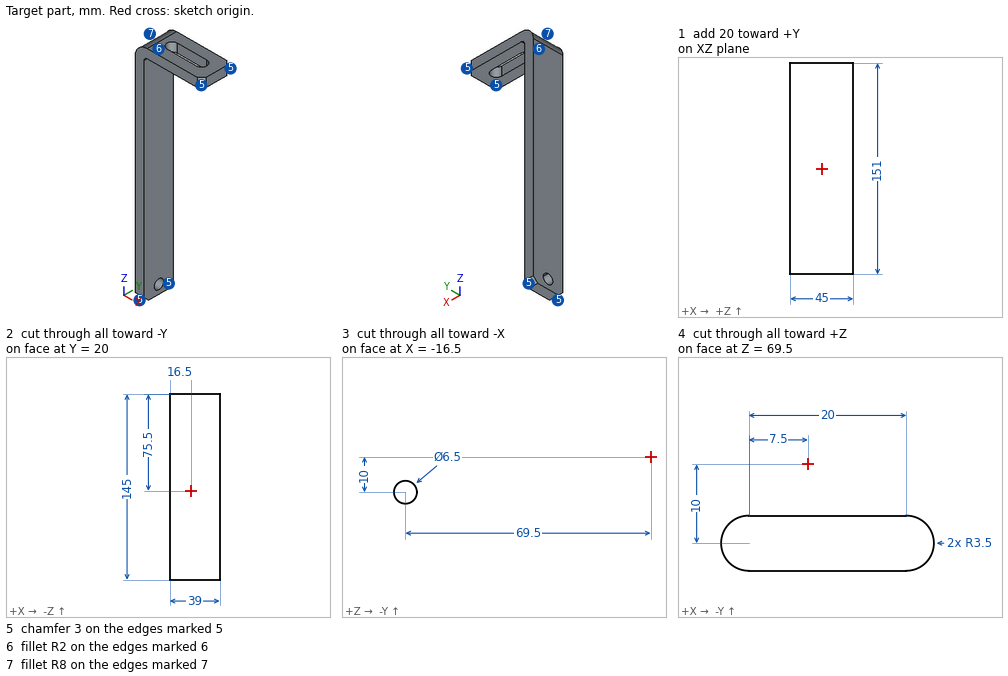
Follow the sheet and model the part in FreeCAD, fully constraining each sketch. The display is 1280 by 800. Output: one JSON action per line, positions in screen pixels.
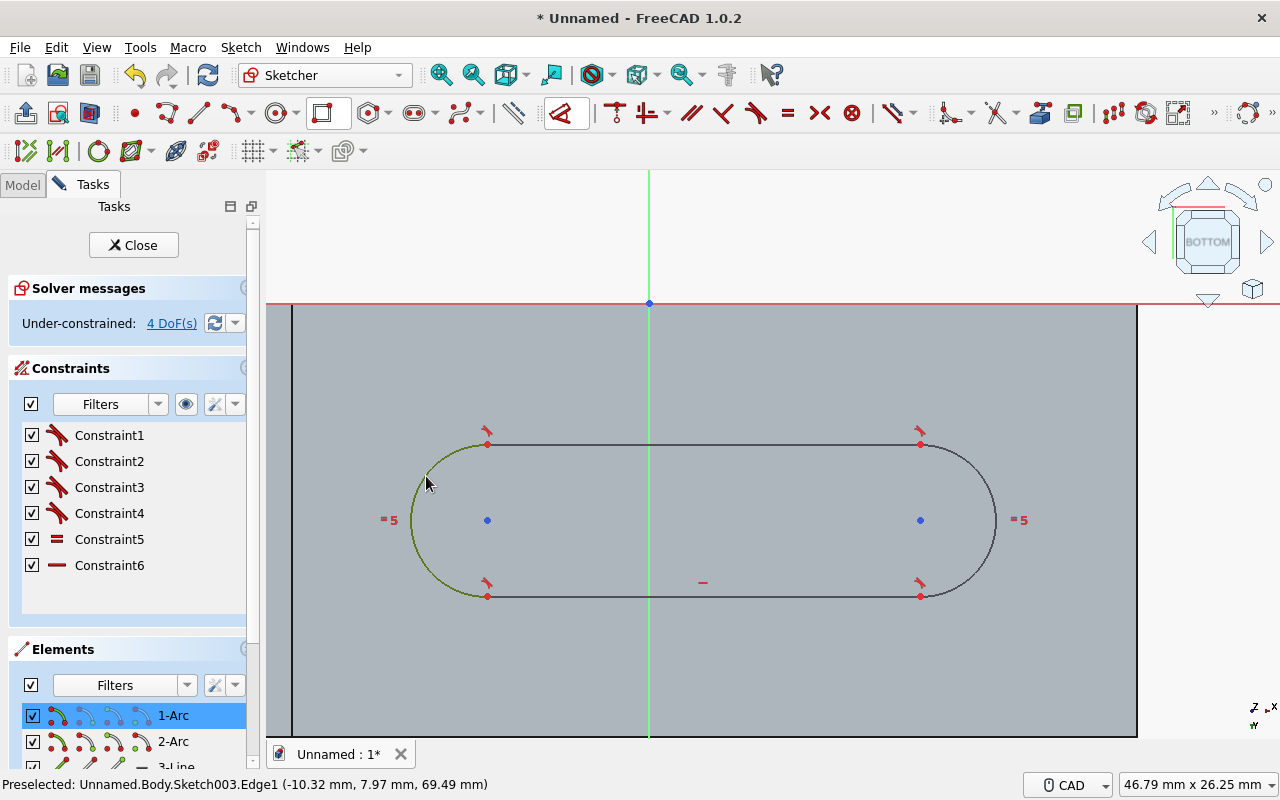
{"action": "key", "text": "k r"}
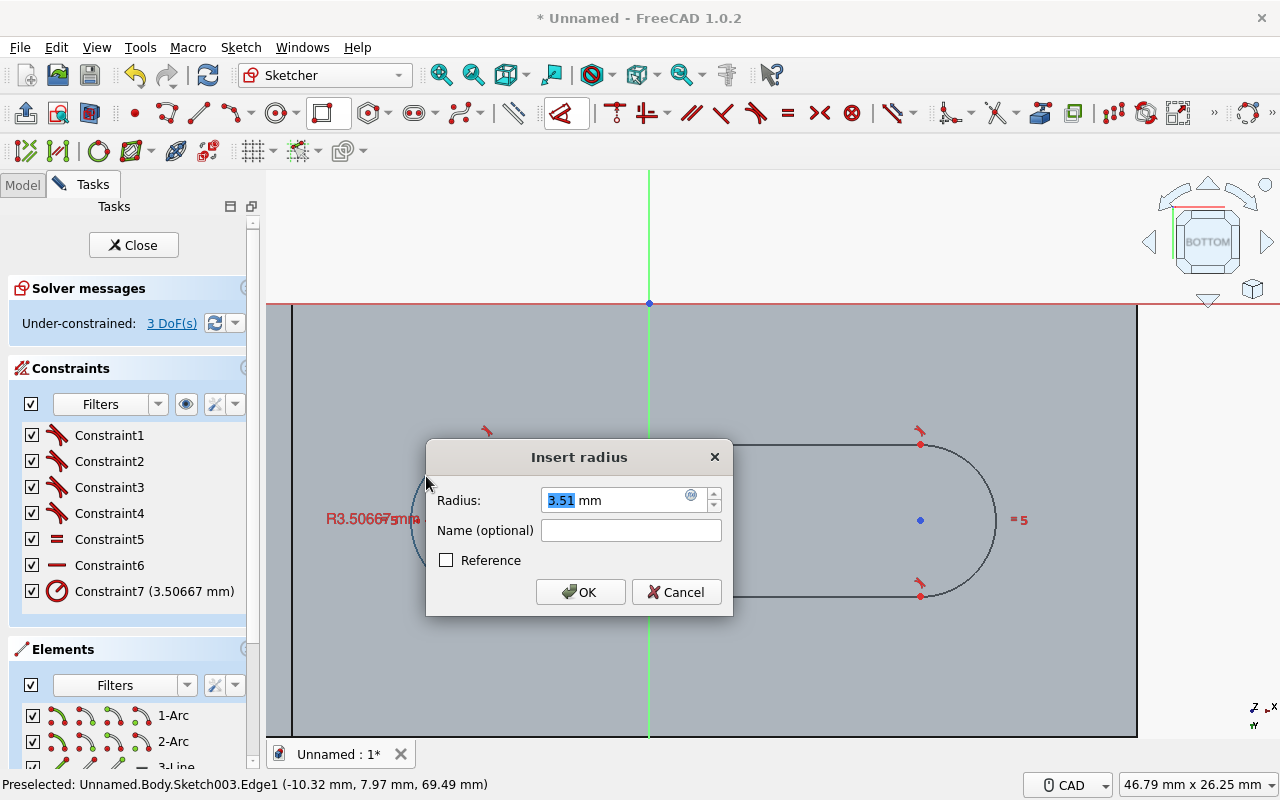
{"action": "type", "text": "3.5"}
{"action": "key", "text": "Return"}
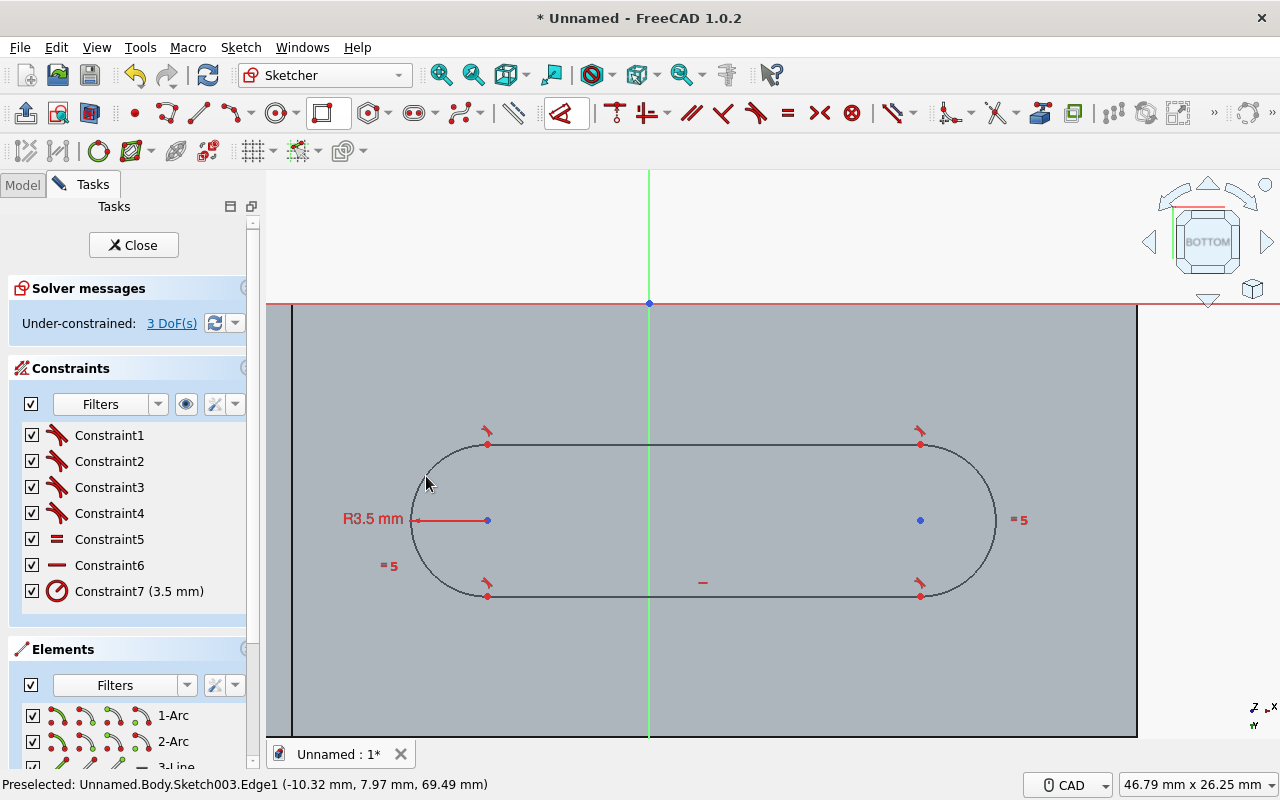
{"action": "left_click", "coordinate": [617, 445]}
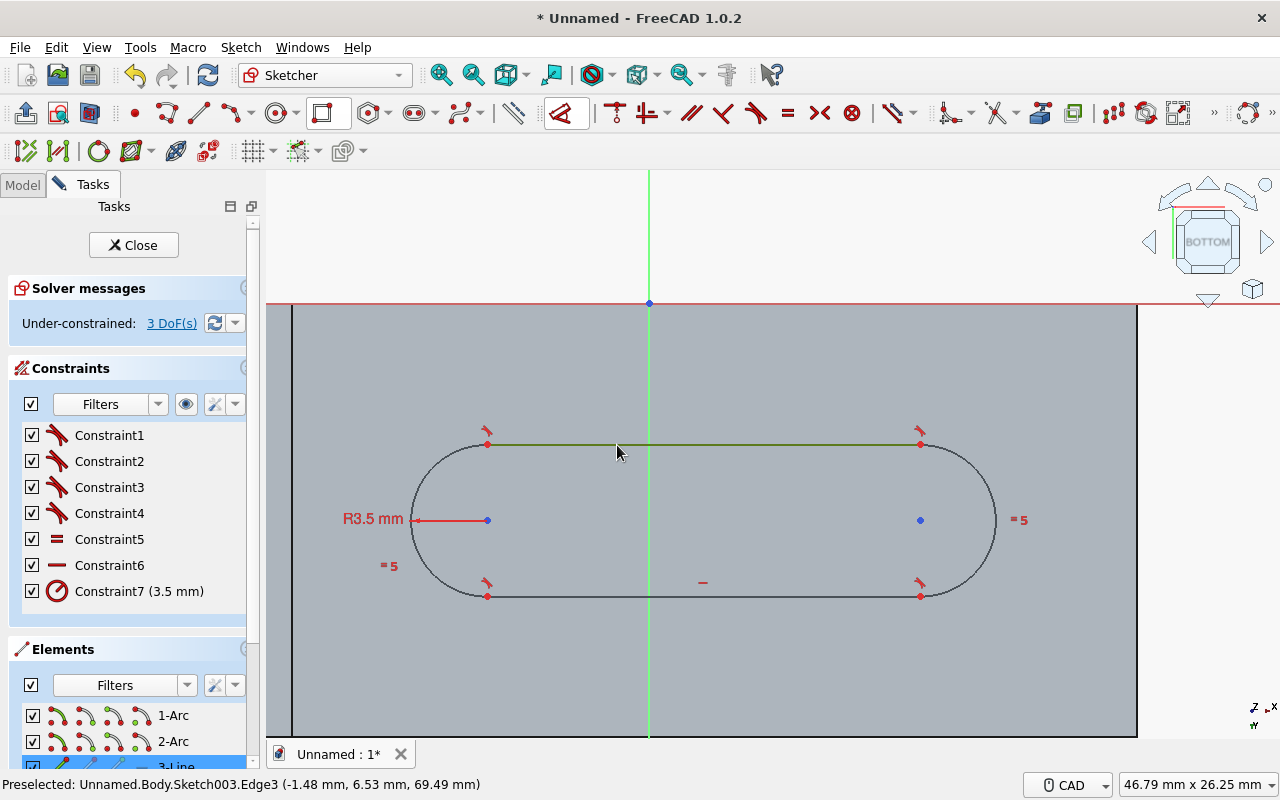
{"action": "key", "text": "l"}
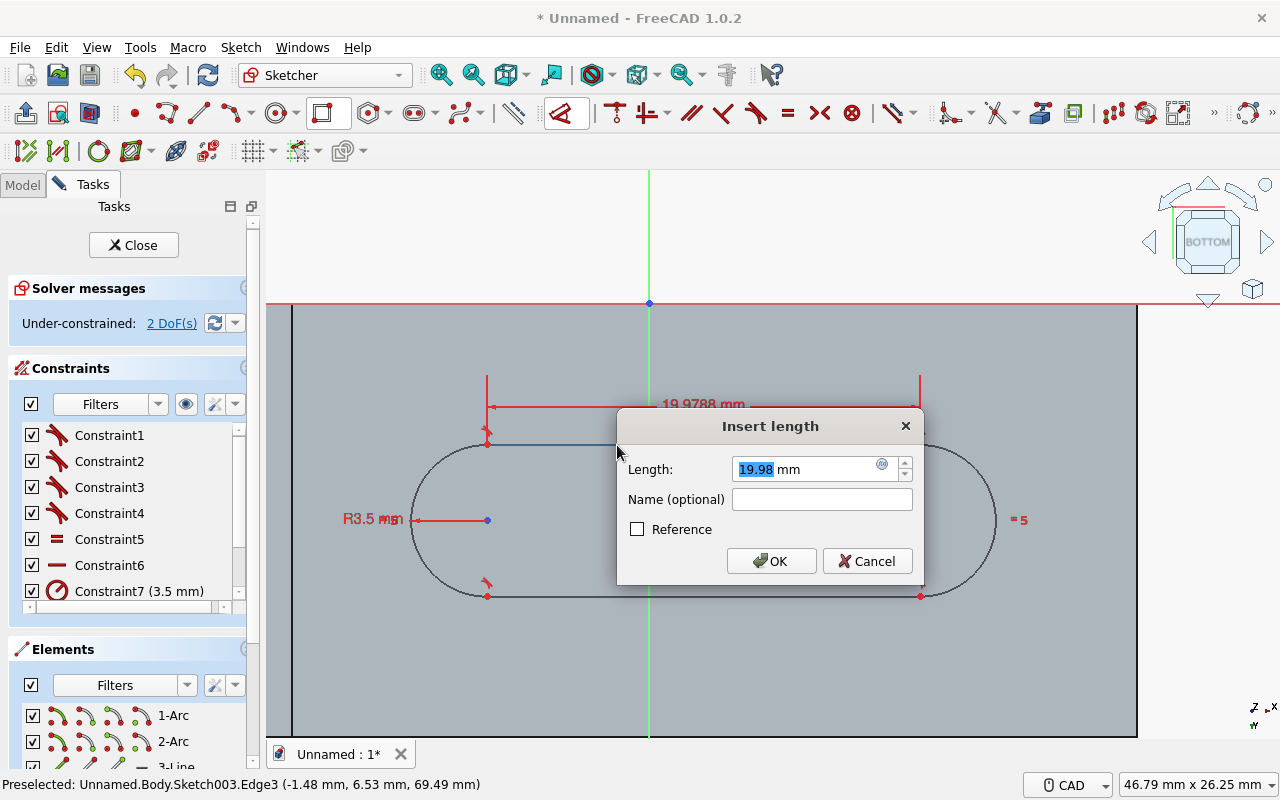
{"action": "type", "text": "20"}
{"action": "key", "text": "Return"}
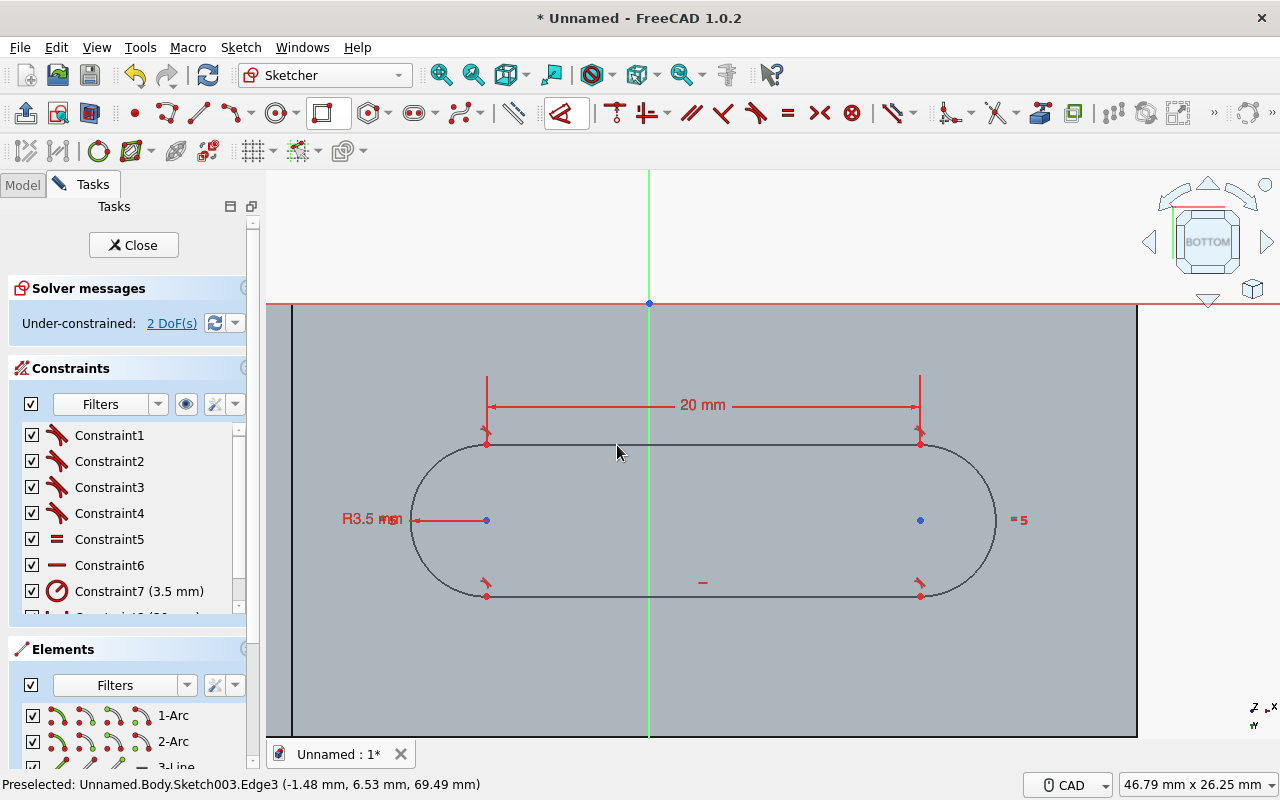
{"action": "left_click", "coordinate": [487, 521]}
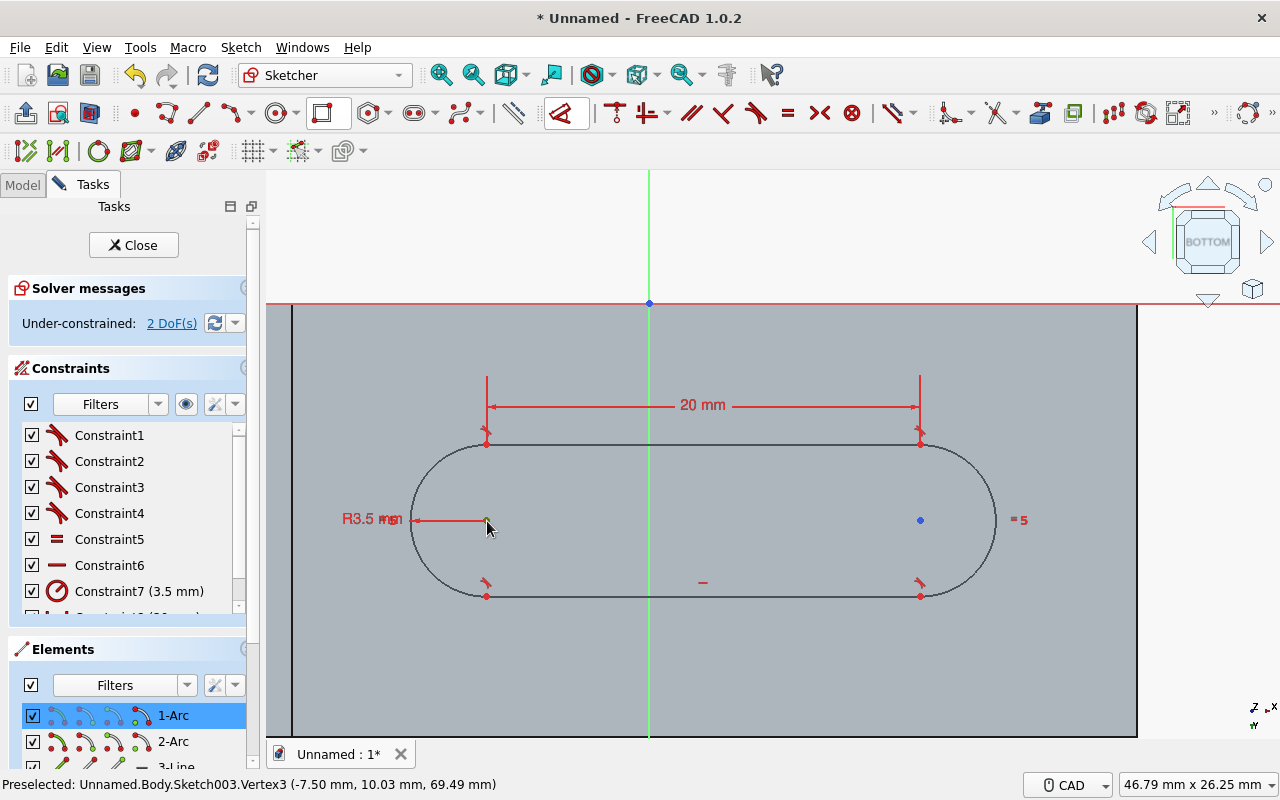
{"action": "left_click", "coordinate": [584, 114]}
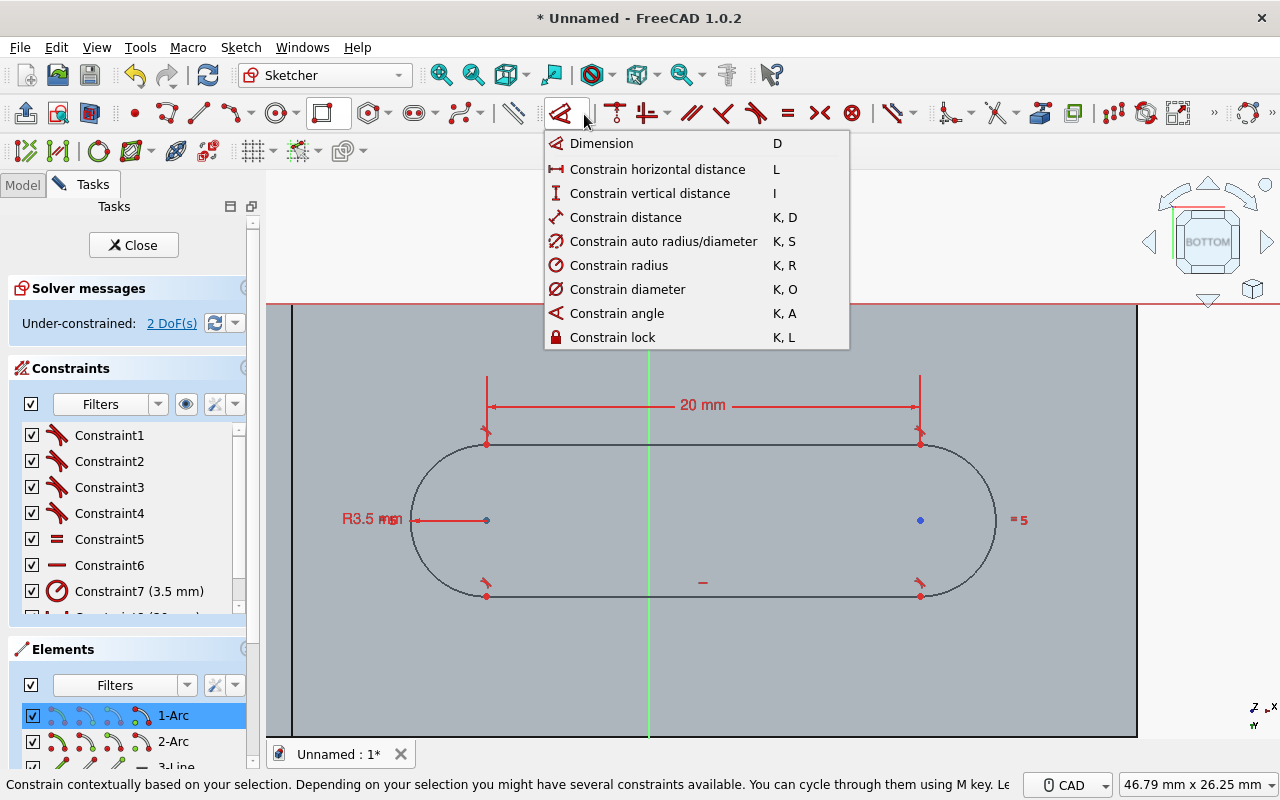
{"action": "left_click", "coordinate": [697, 193]}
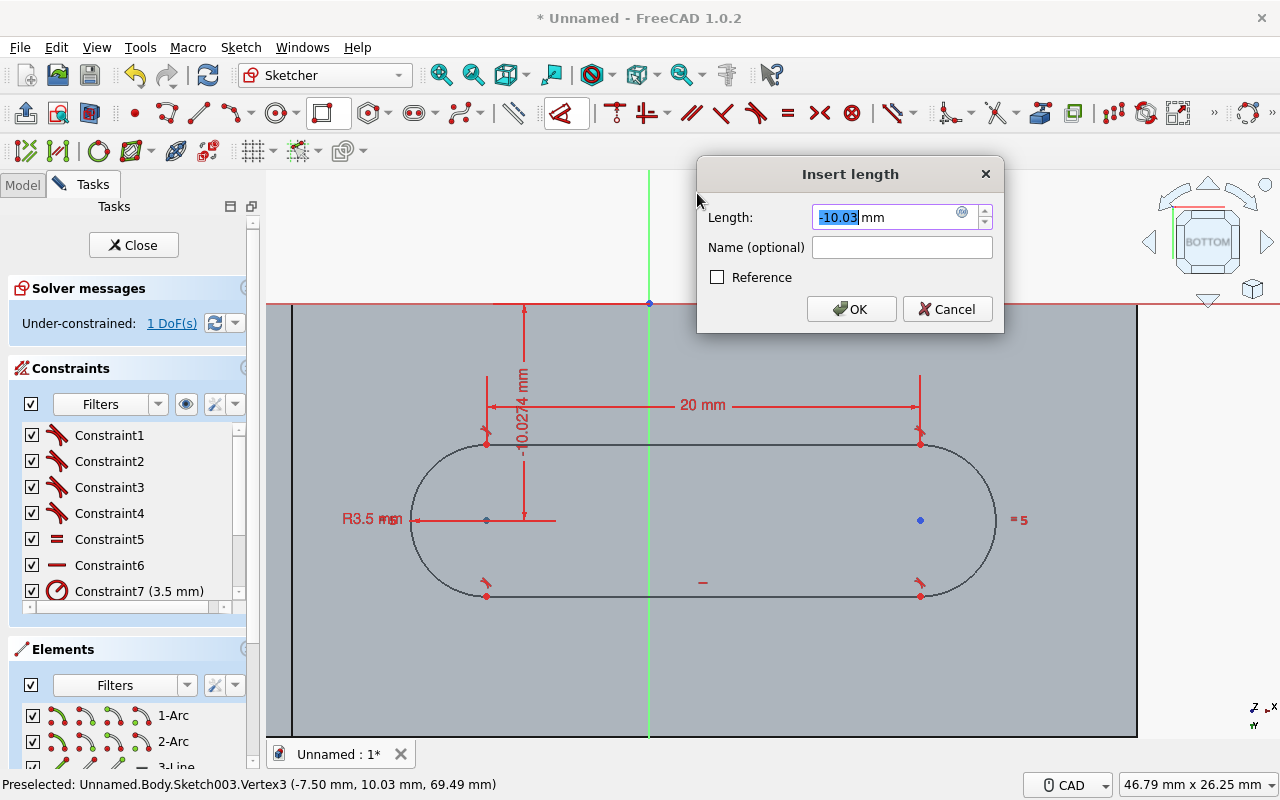
{"action": "type", "text": "-10"}
{"action": "key", "text": "Return"}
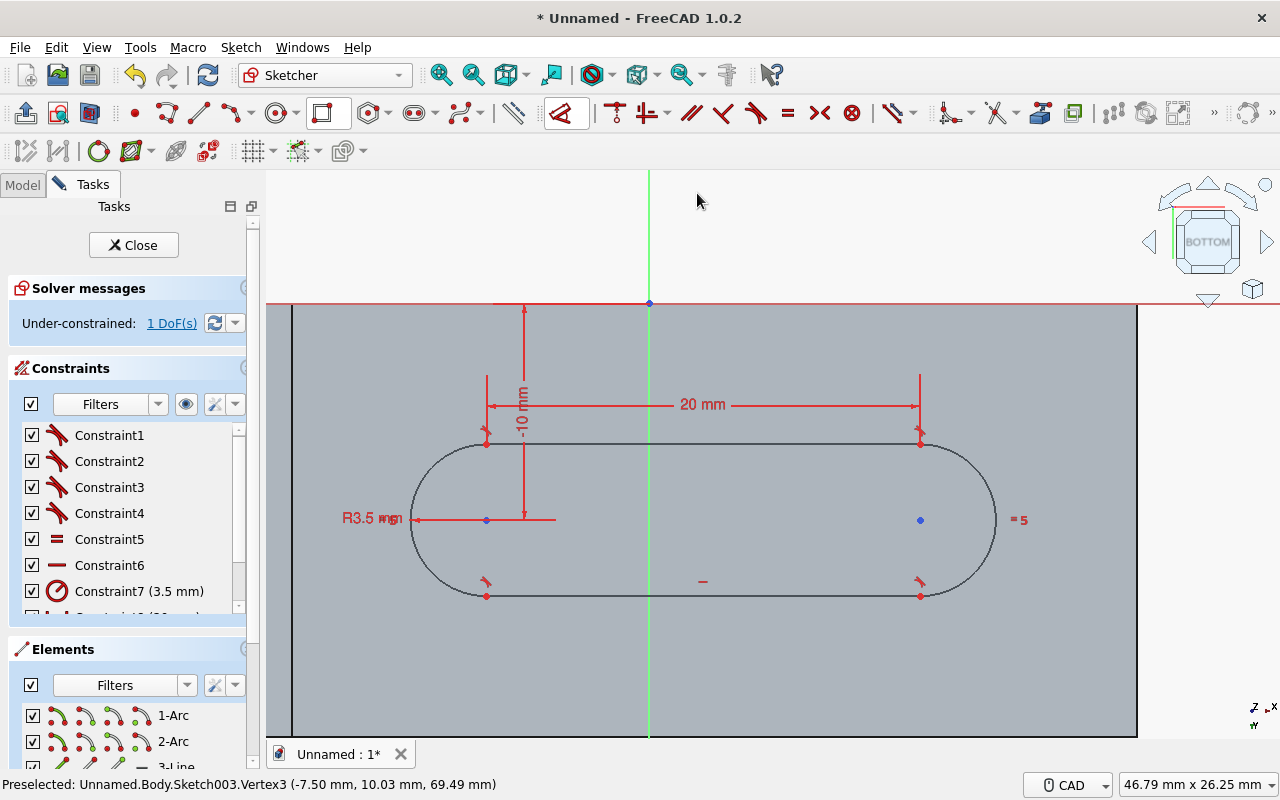
{"action": "left_click", "coordinate": [487, 444]}